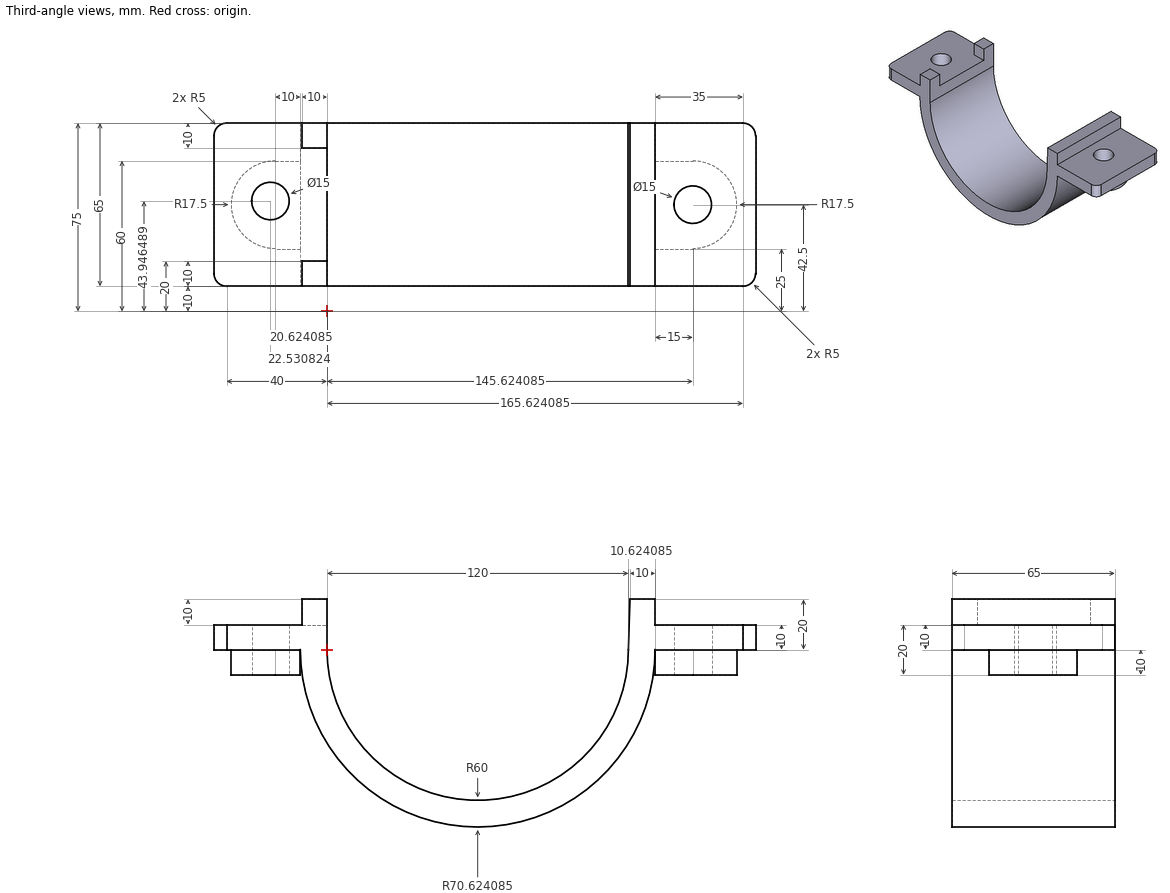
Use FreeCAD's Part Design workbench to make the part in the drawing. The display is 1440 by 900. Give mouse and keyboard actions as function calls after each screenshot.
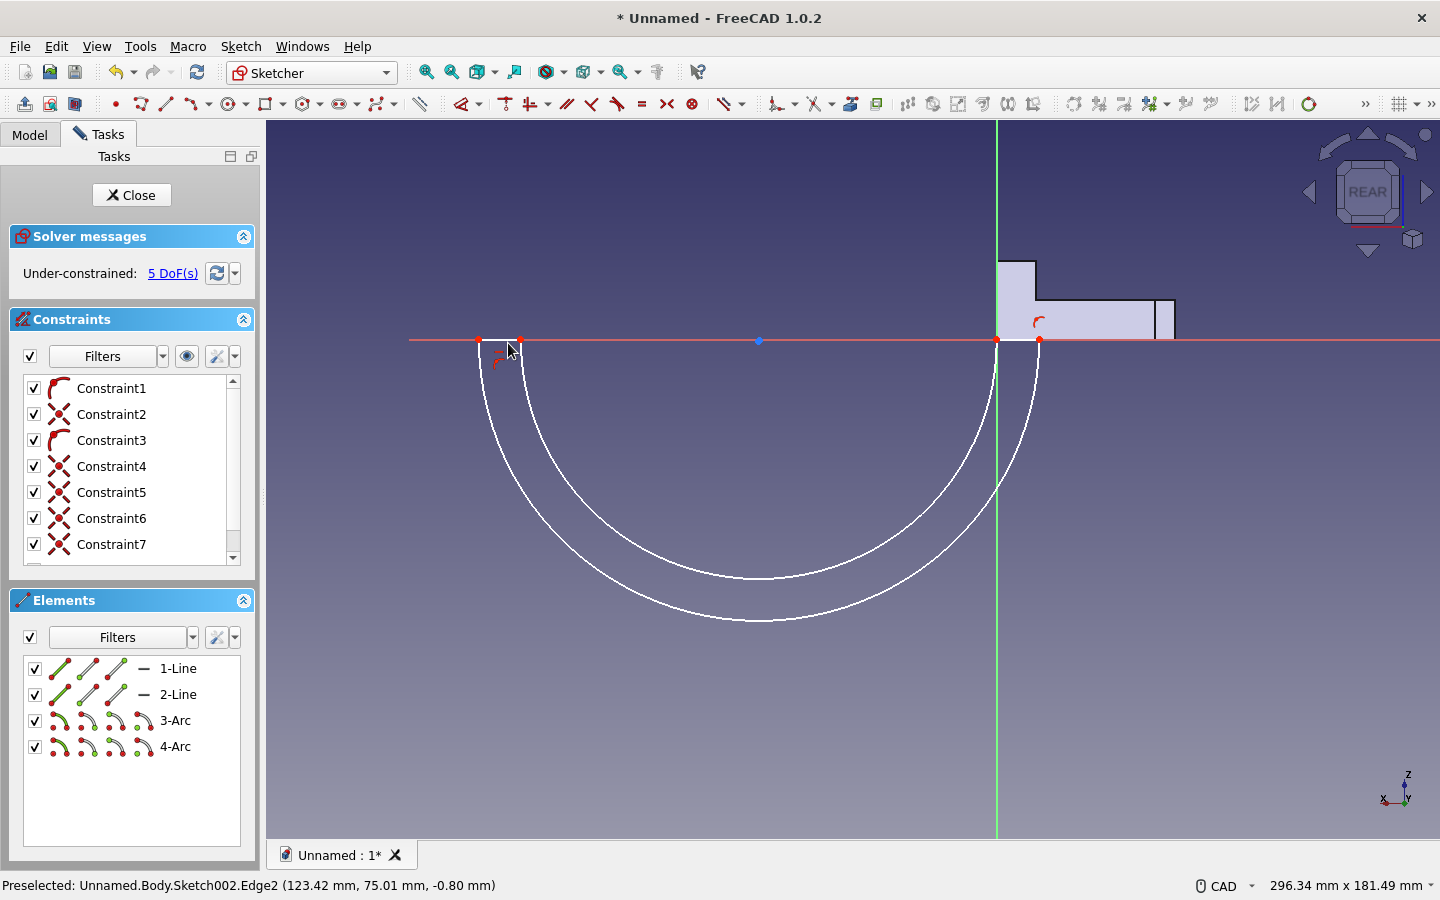
click(619, 533)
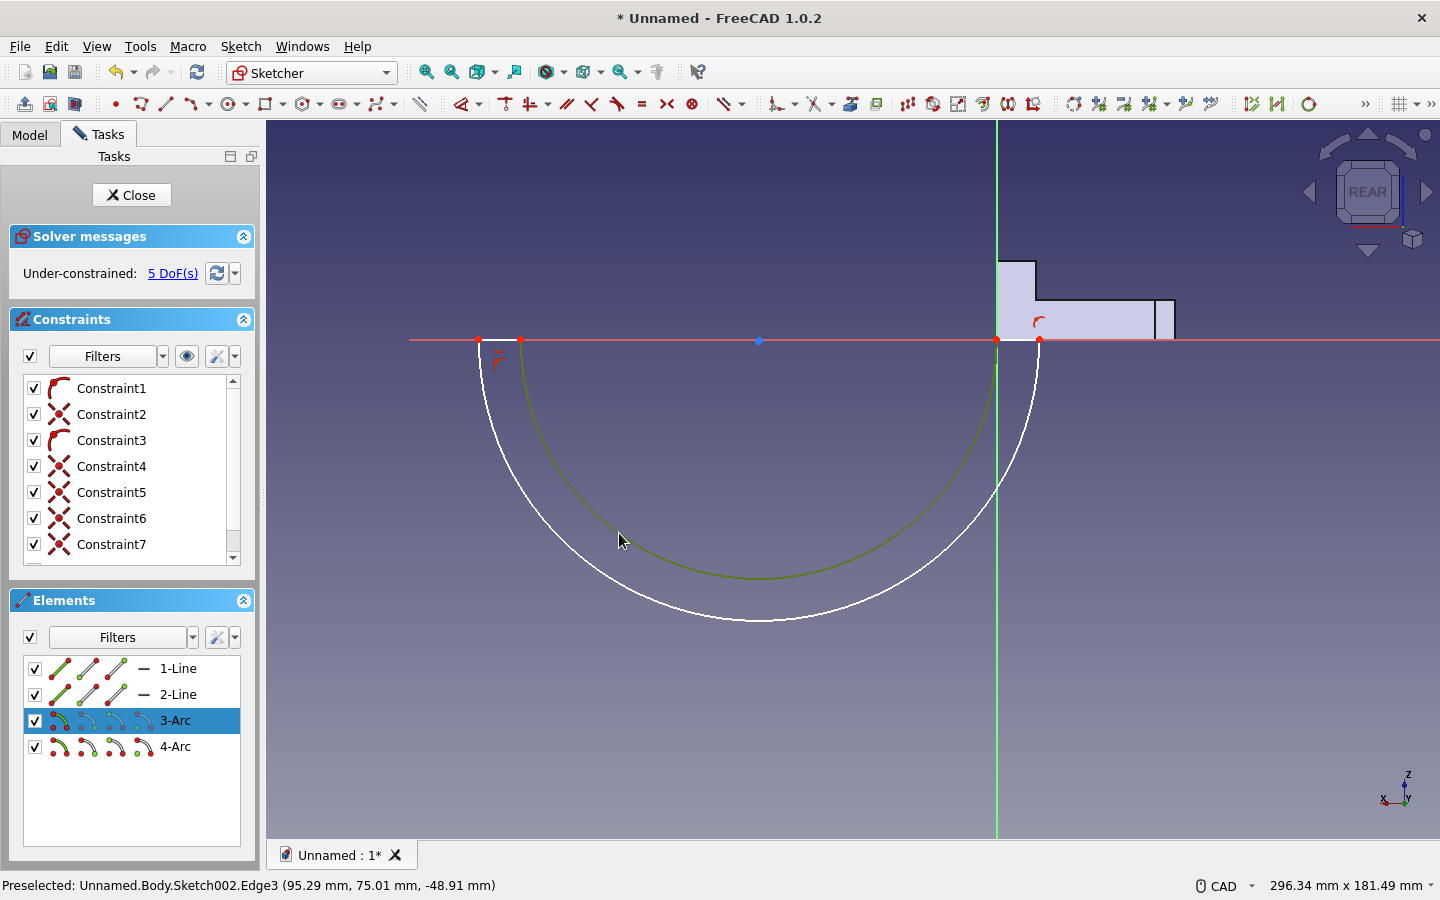
click(594, 567)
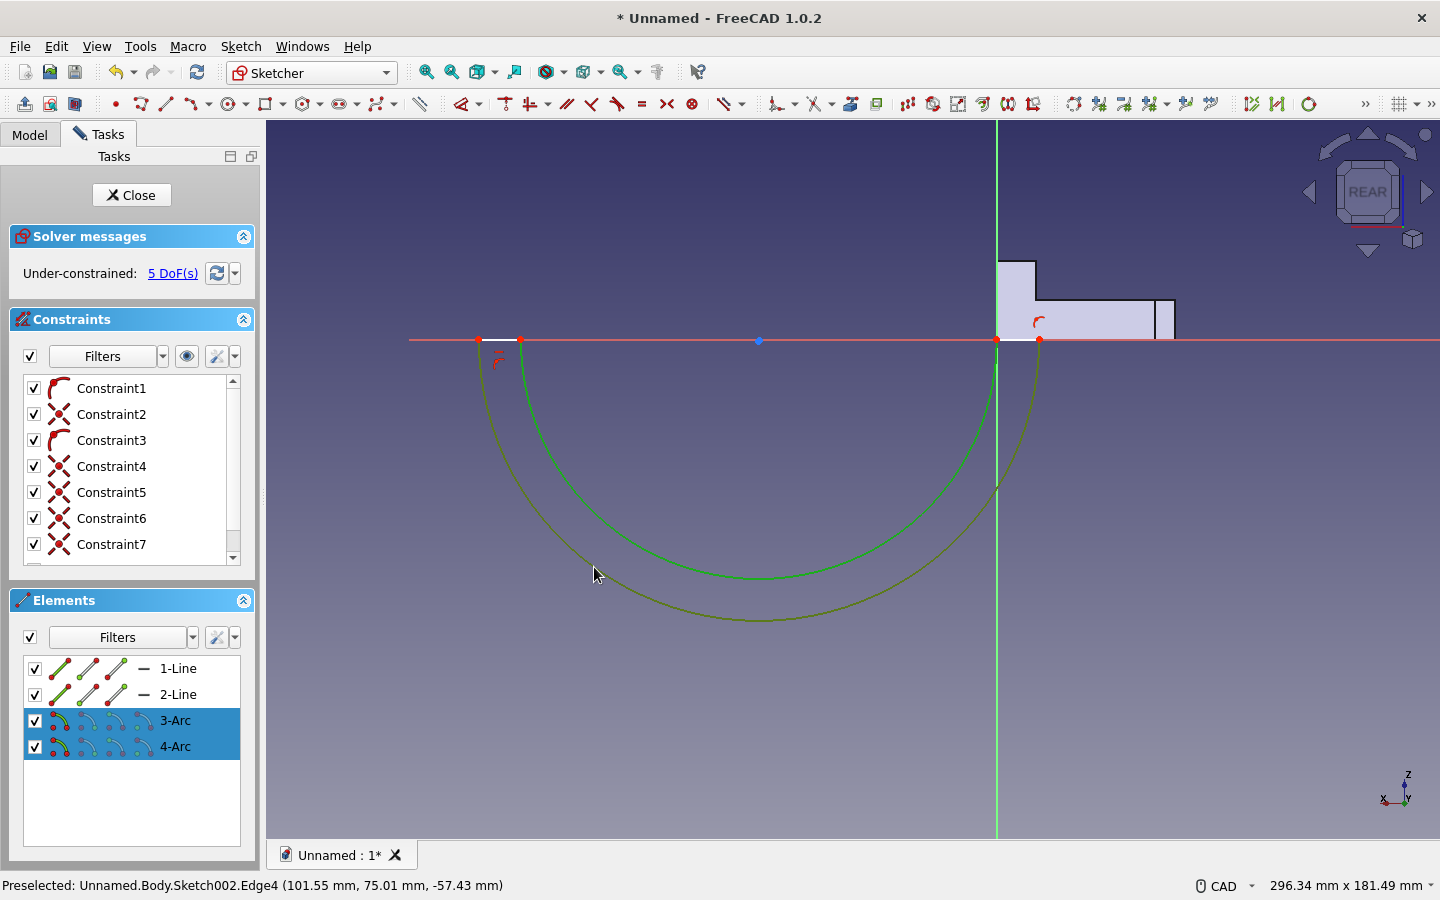
key(c)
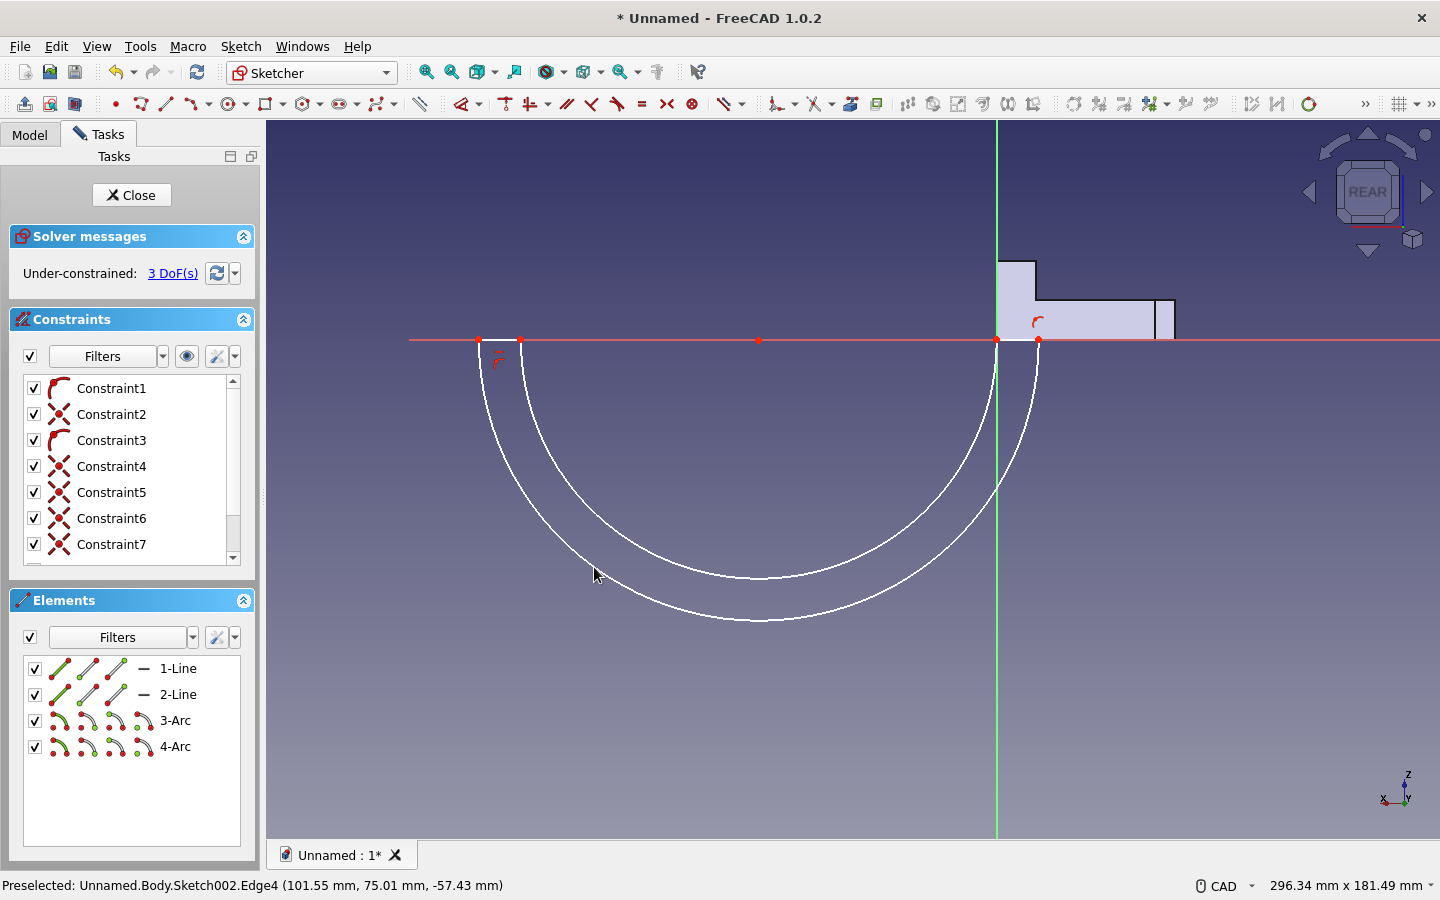
click(759, 341)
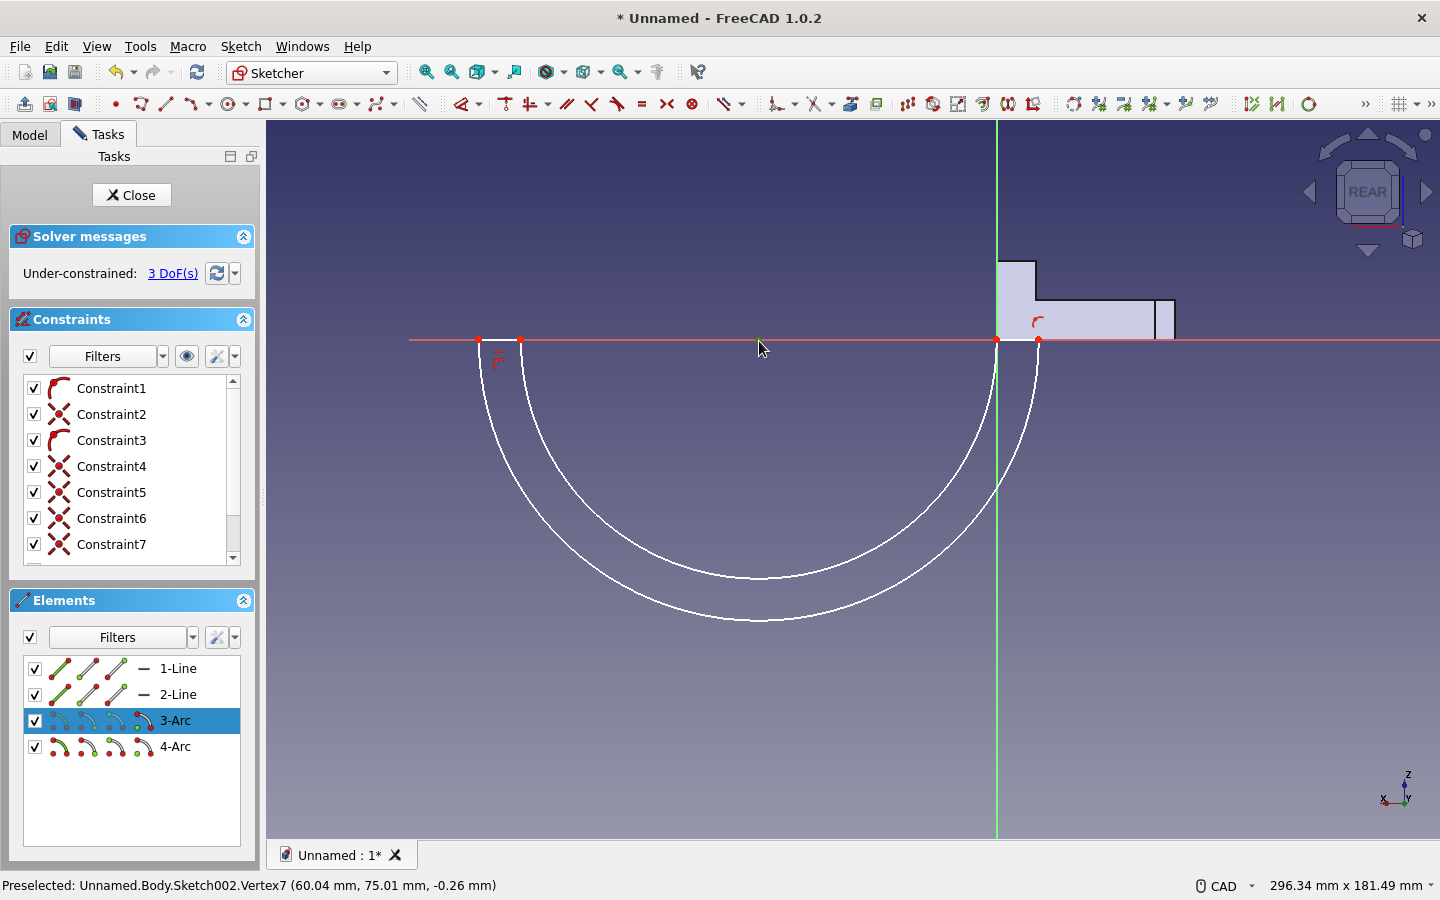
click(434, 340)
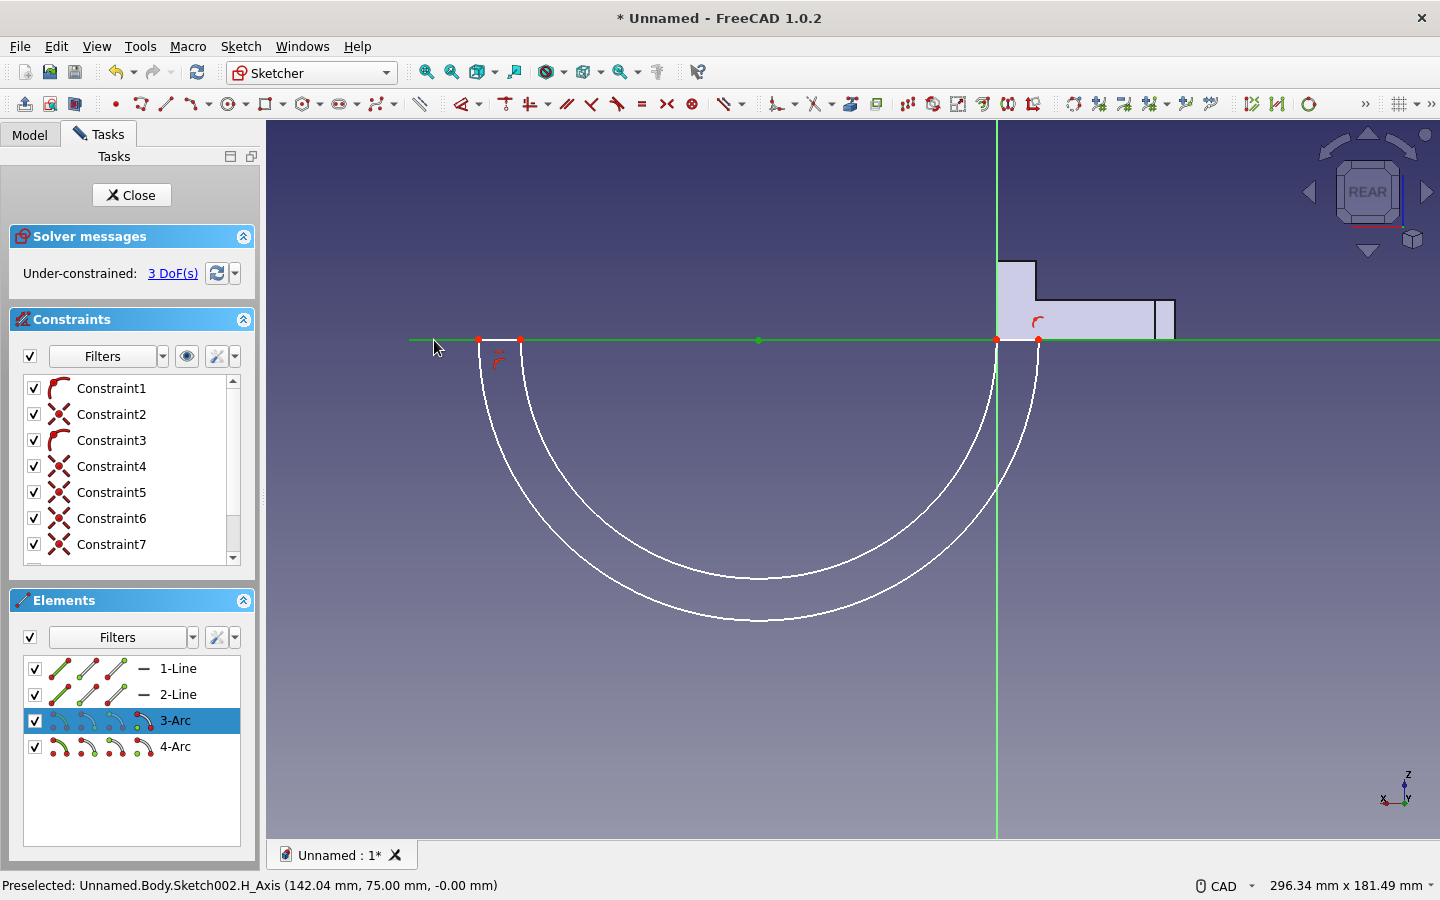
key(c)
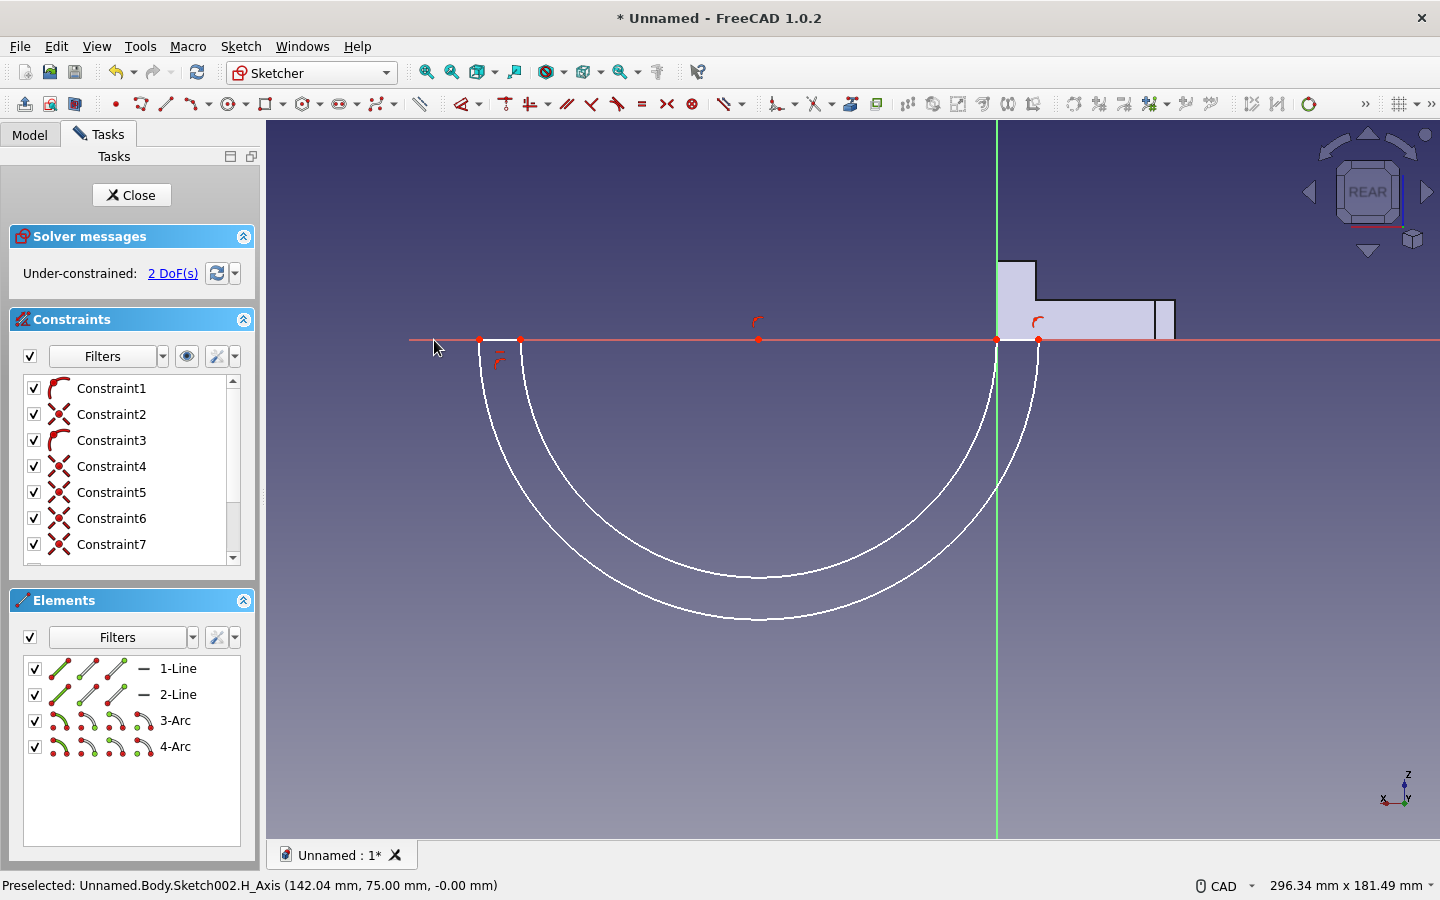
click(460, 104)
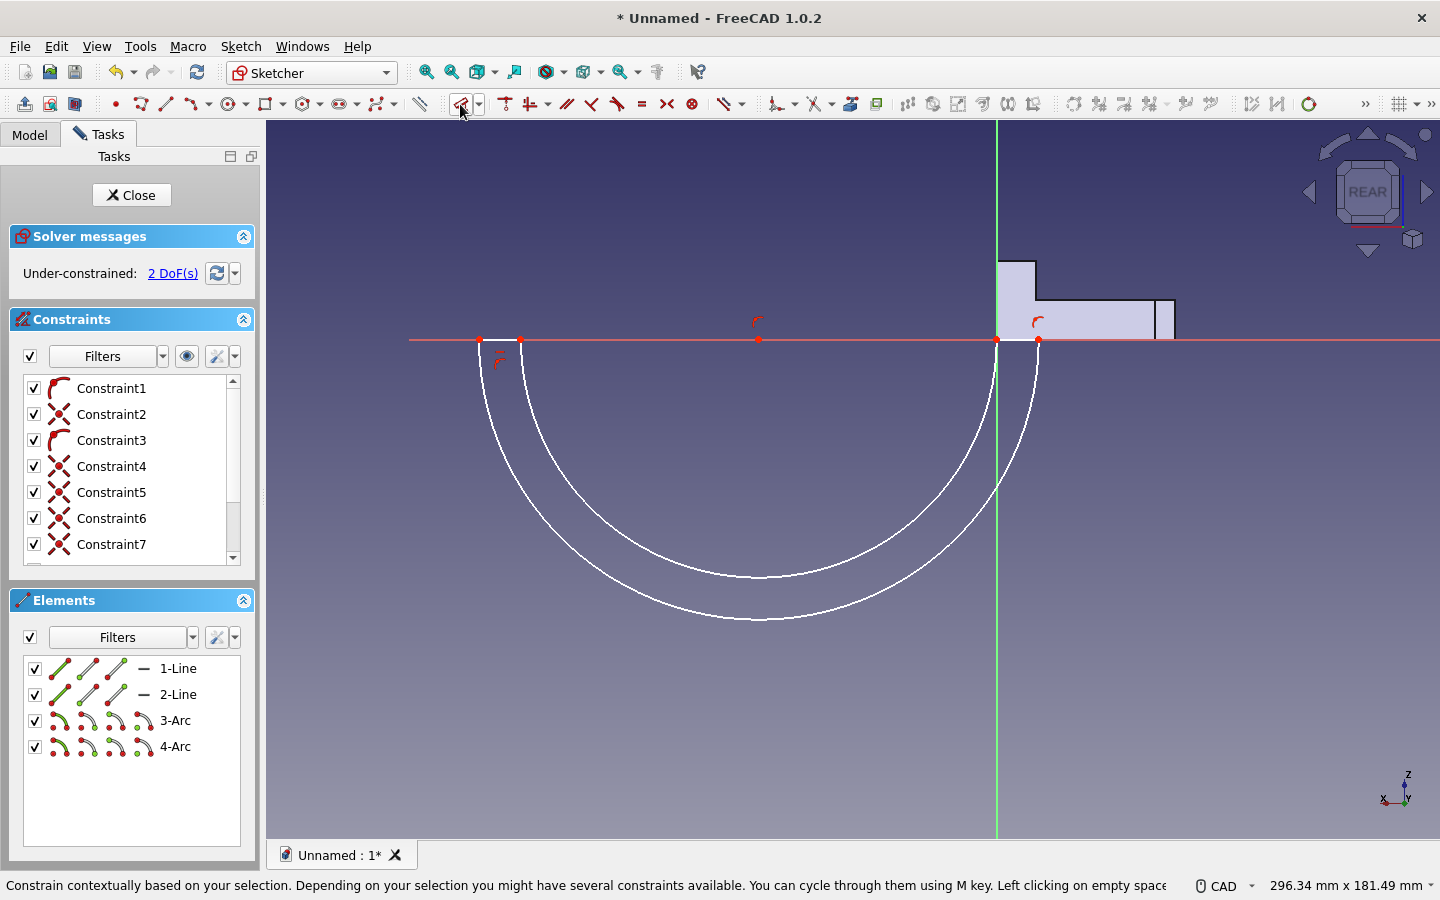
click(619, 532)
click(490, 324)